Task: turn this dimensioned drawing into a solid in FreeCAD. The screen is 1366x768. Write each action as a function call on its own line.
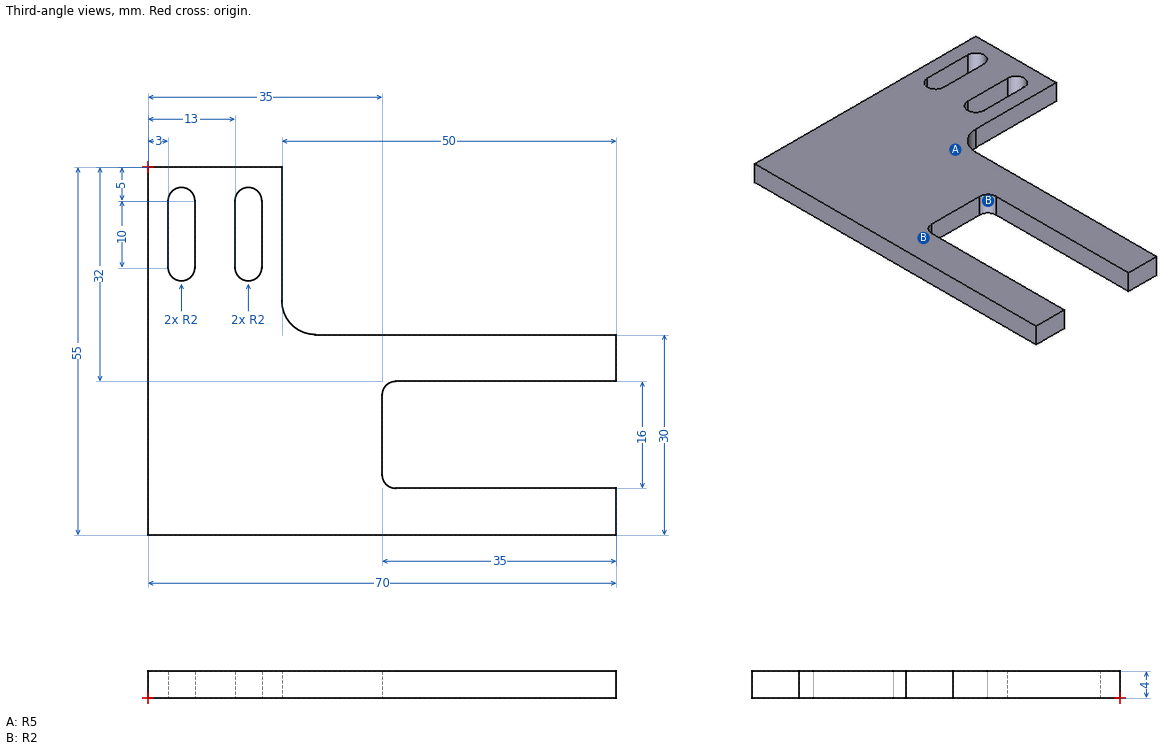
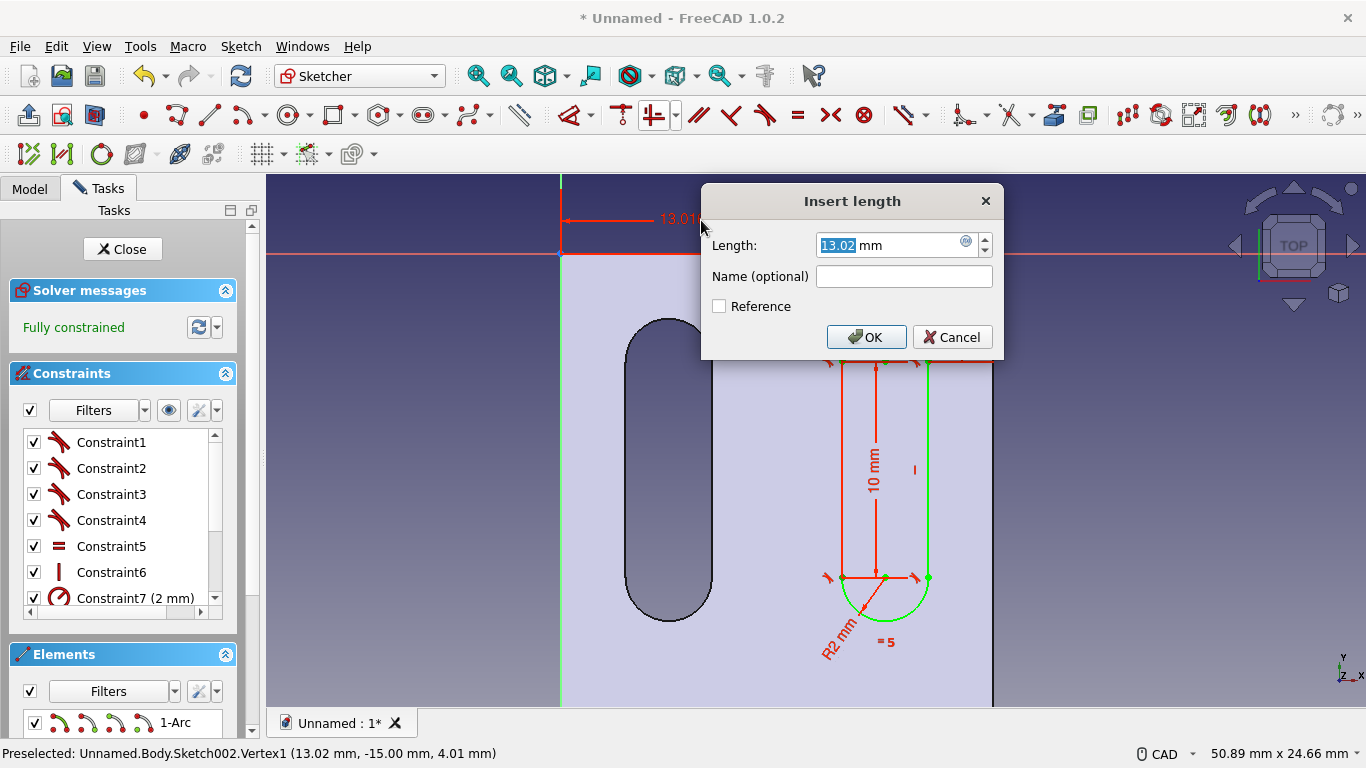
text(13)
key(Return)
key(Escape)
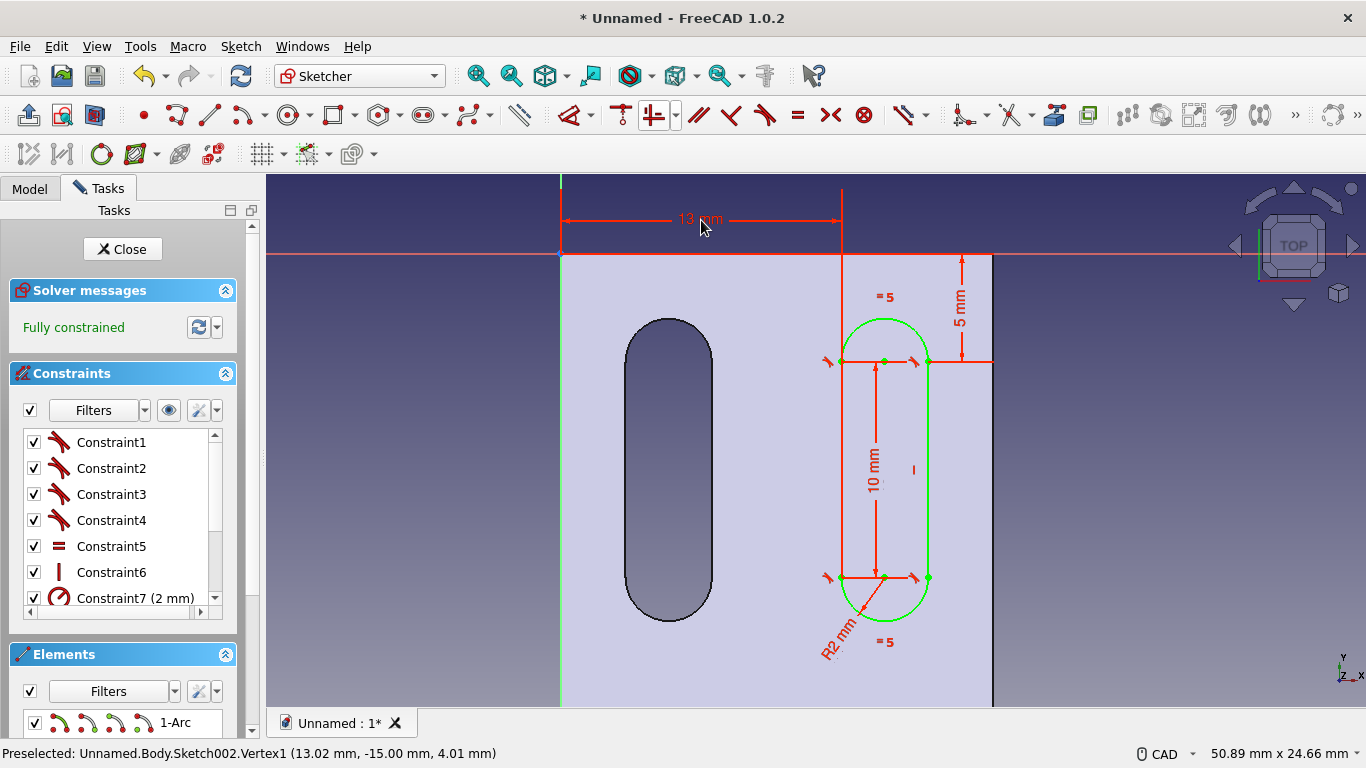
click(123, 249)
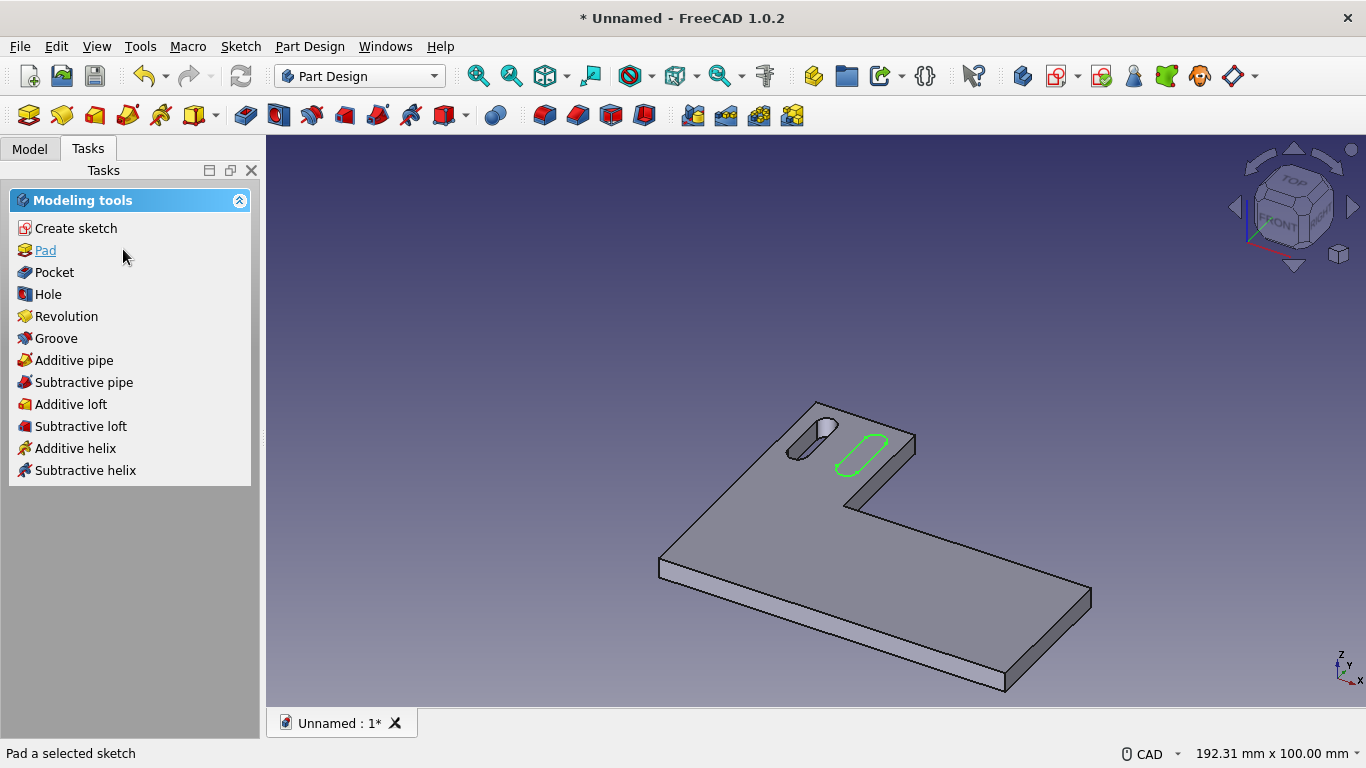
click(246, 116)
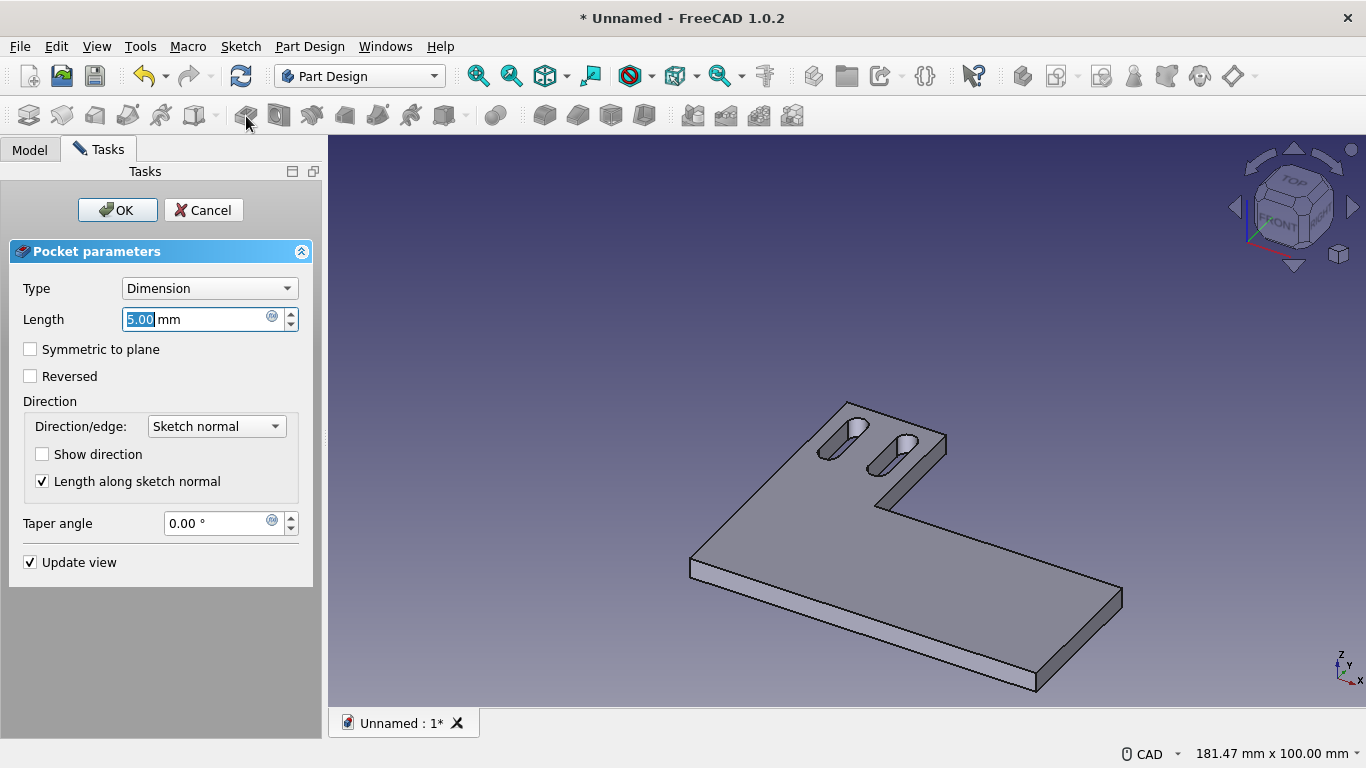
click(210, 288)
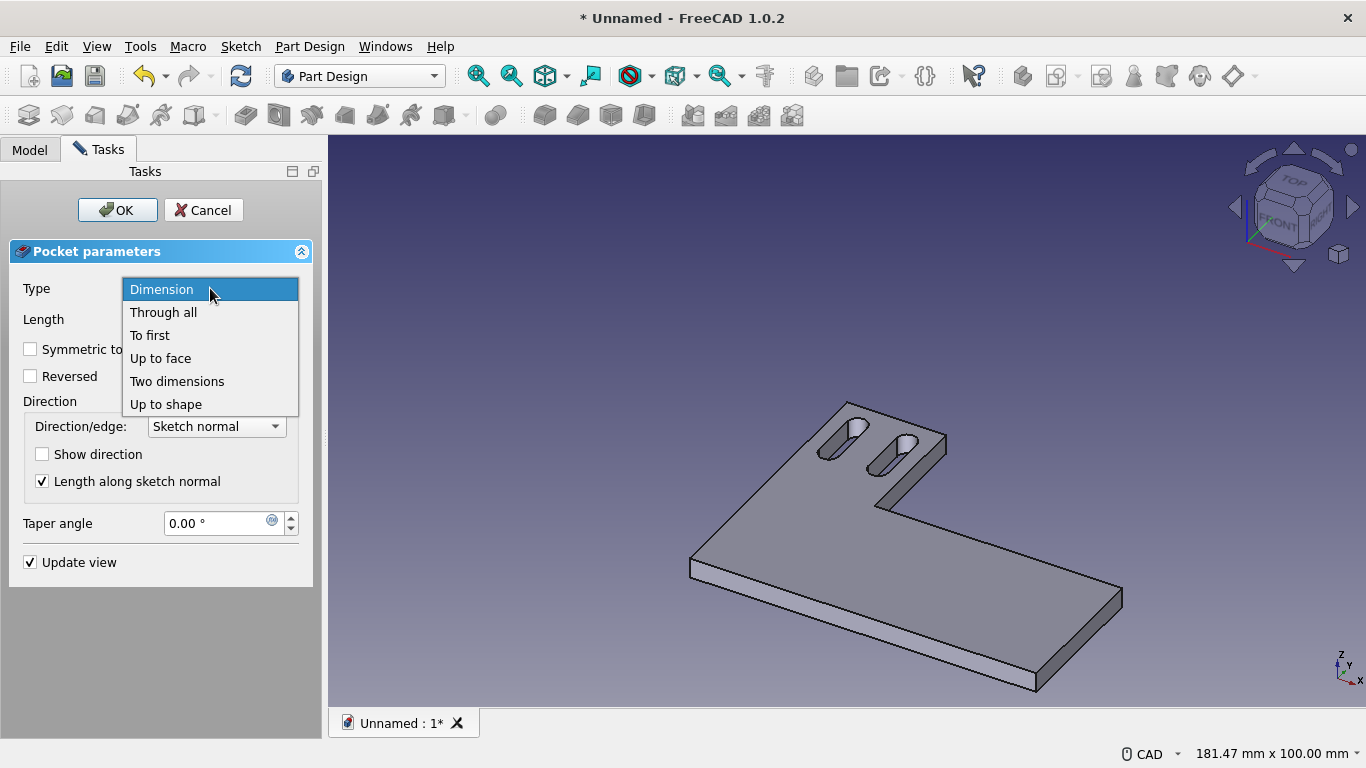
click(208, 336)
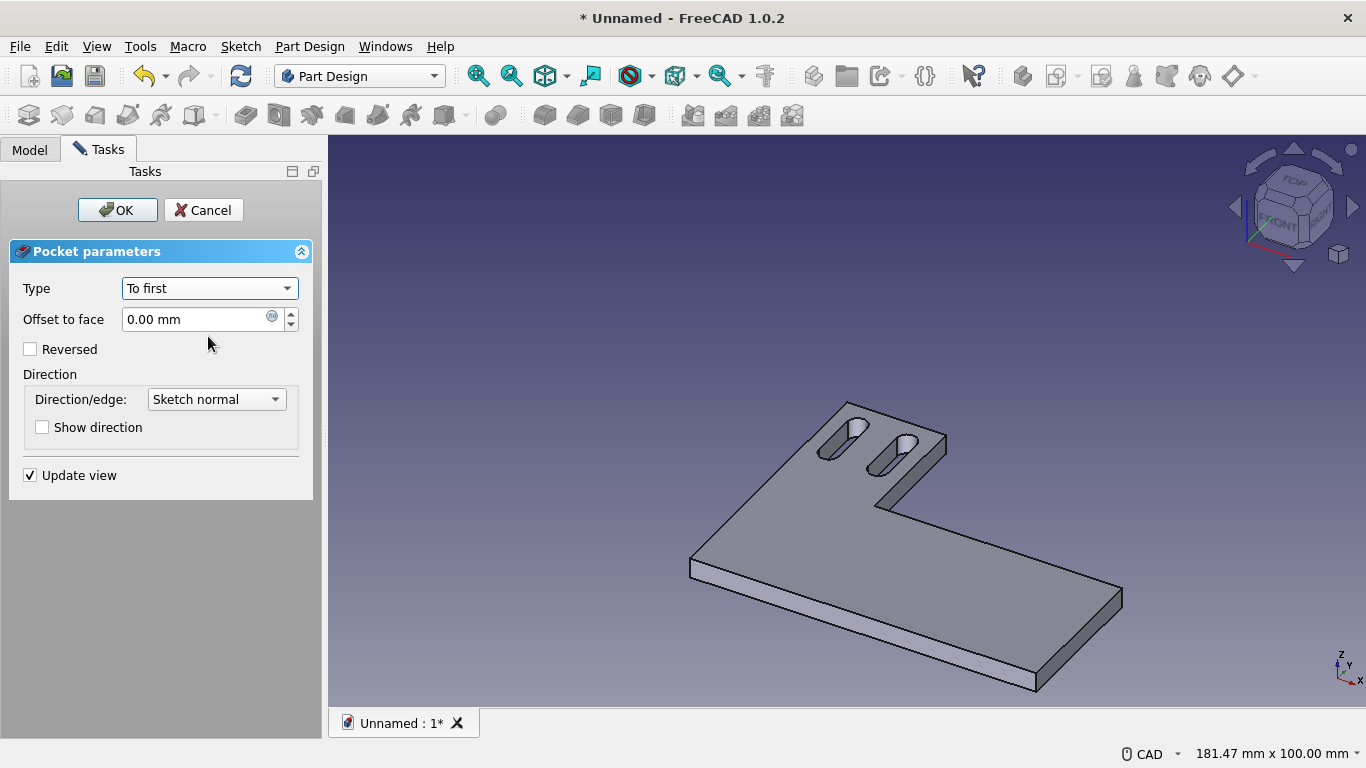
click(118, 210)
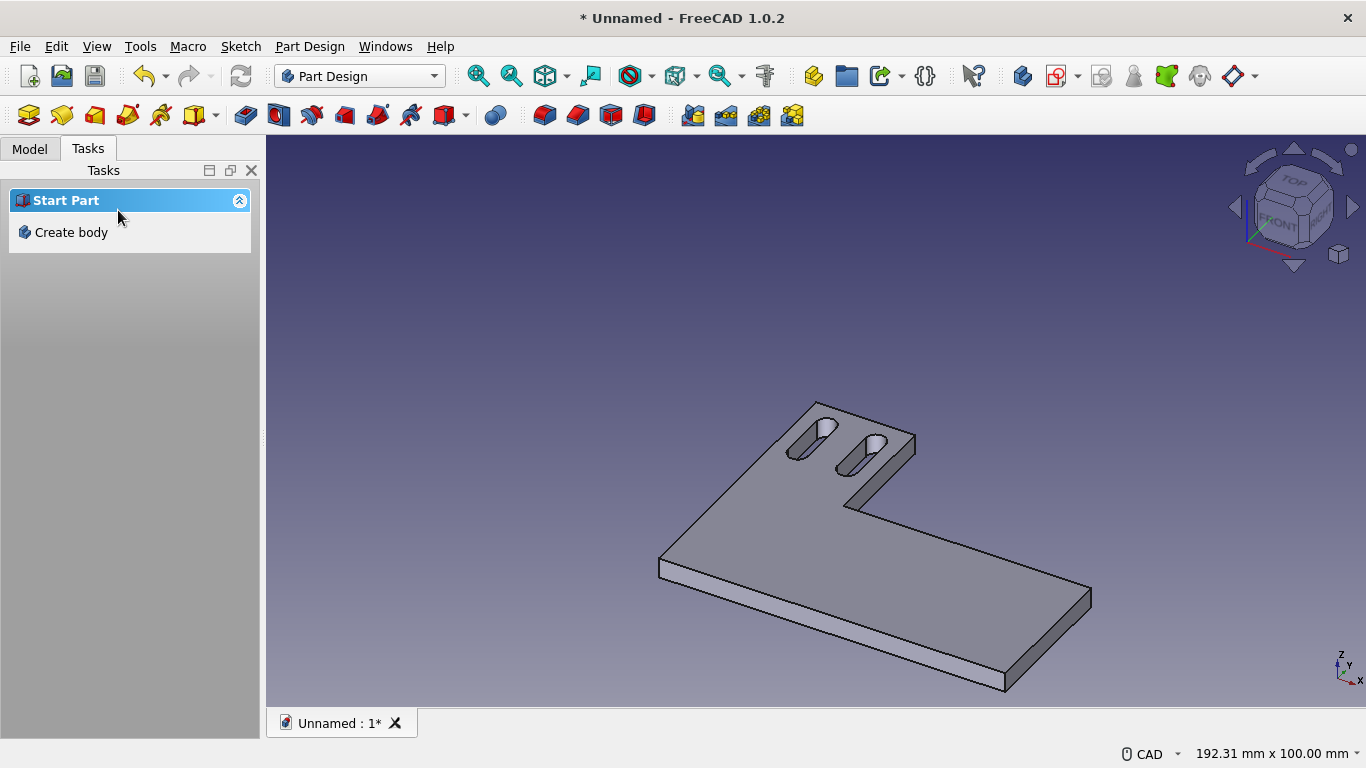
key(0)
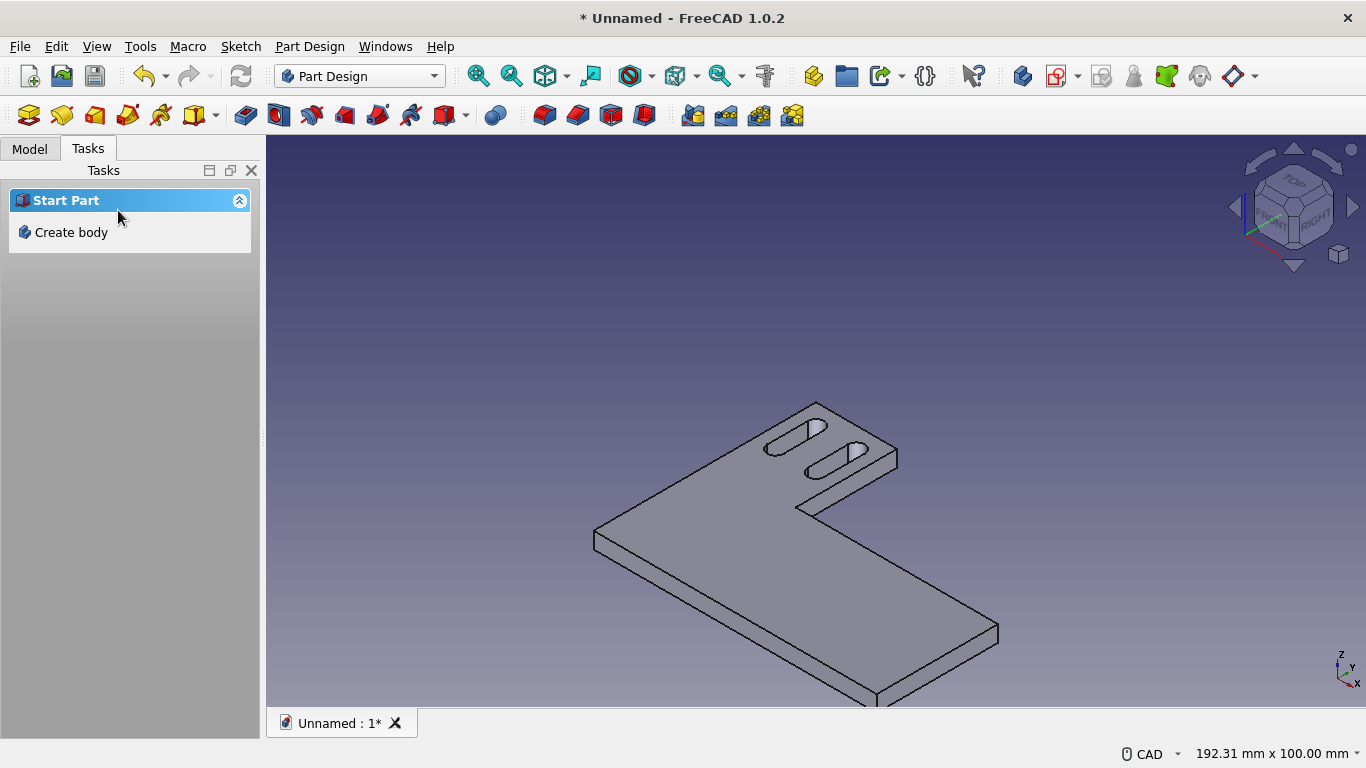
click(479, 76)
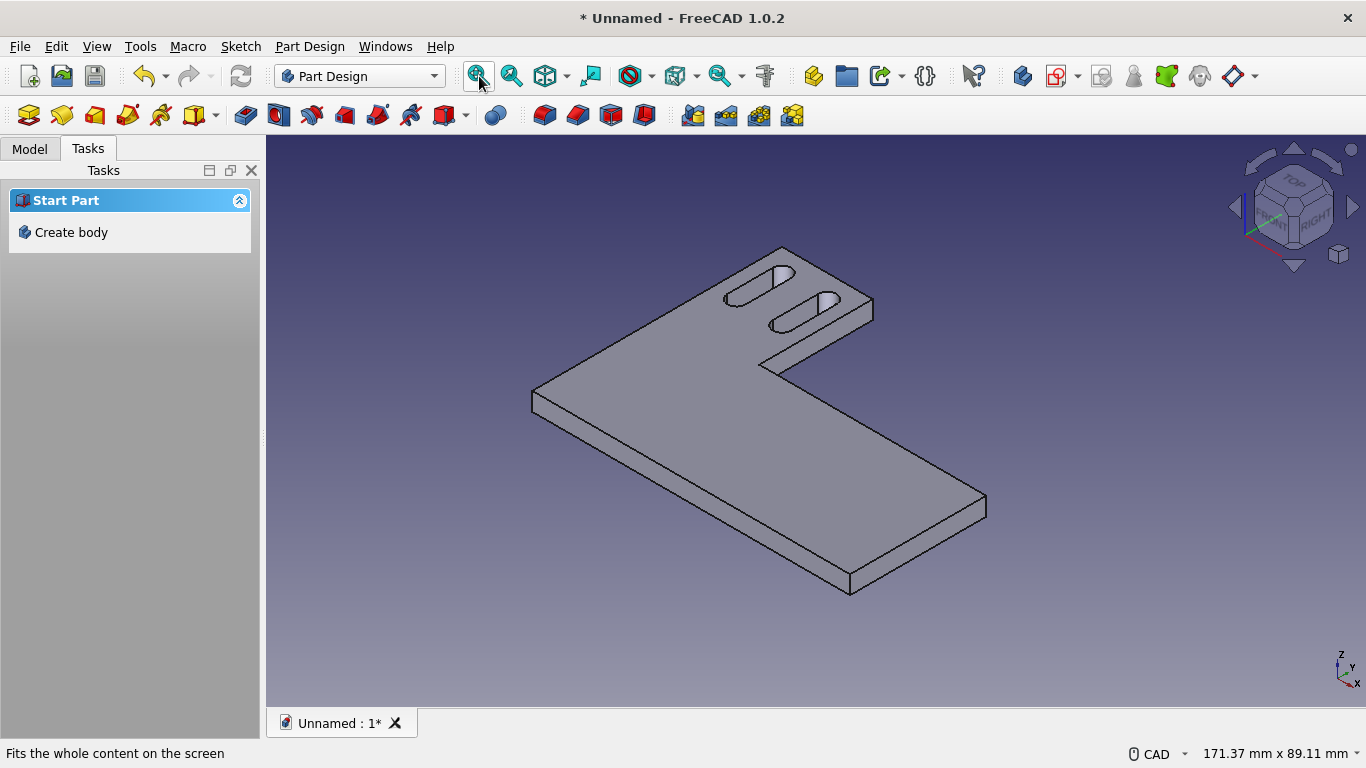
key(2)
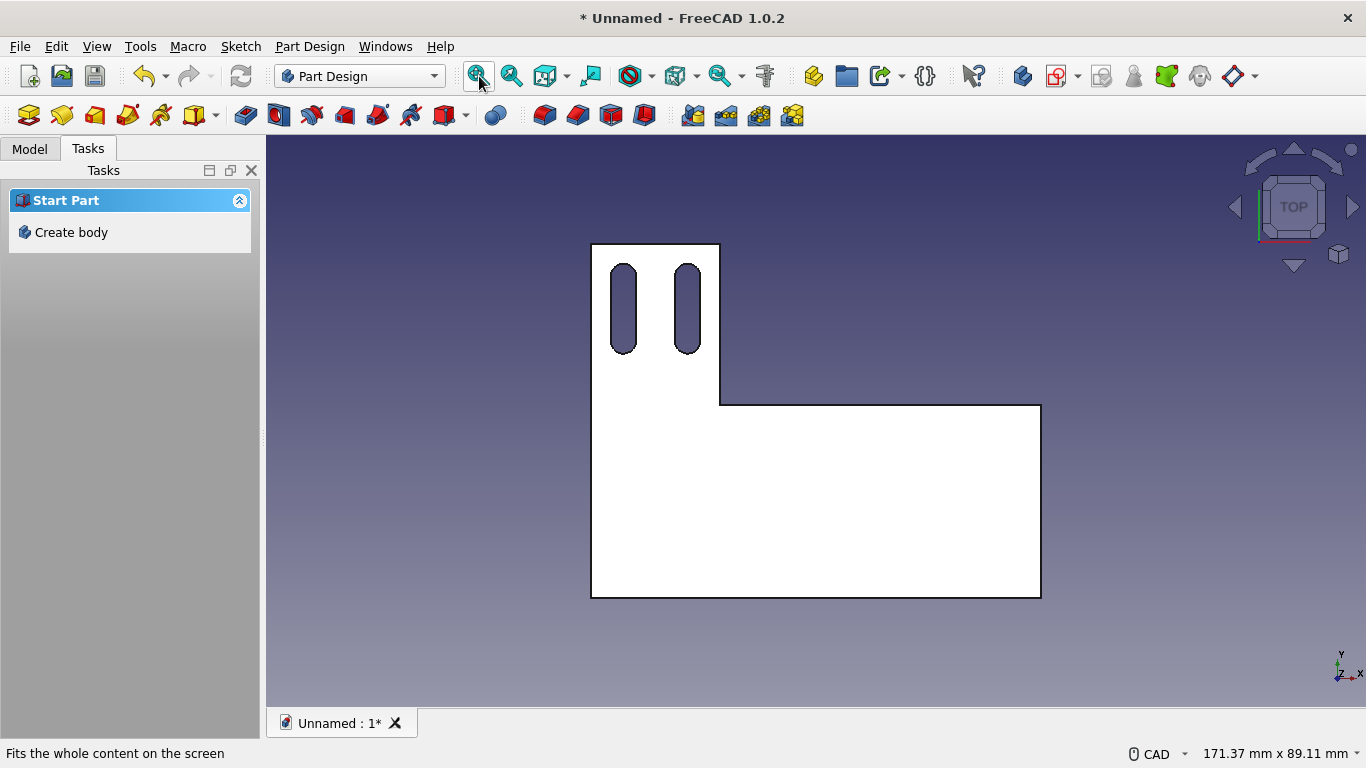
key(1)